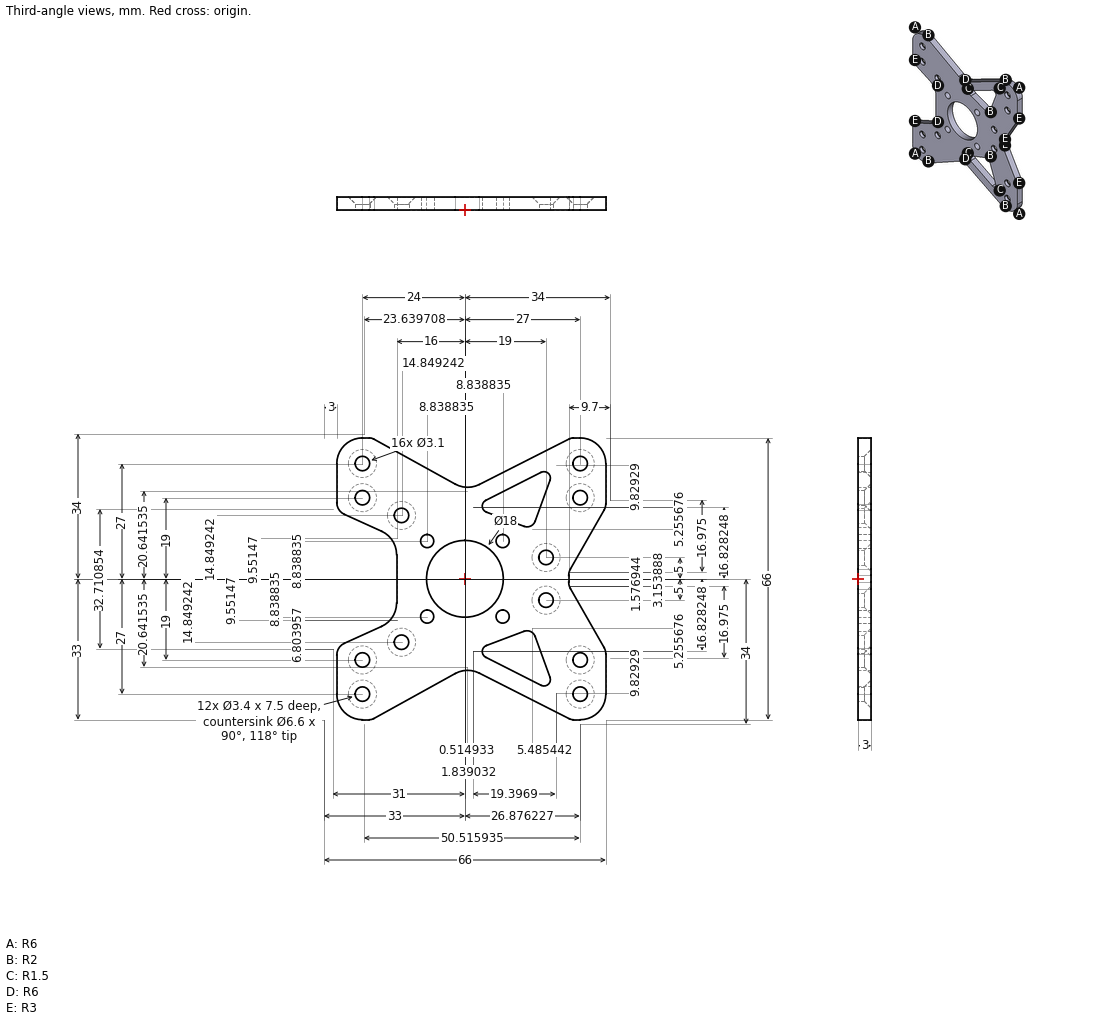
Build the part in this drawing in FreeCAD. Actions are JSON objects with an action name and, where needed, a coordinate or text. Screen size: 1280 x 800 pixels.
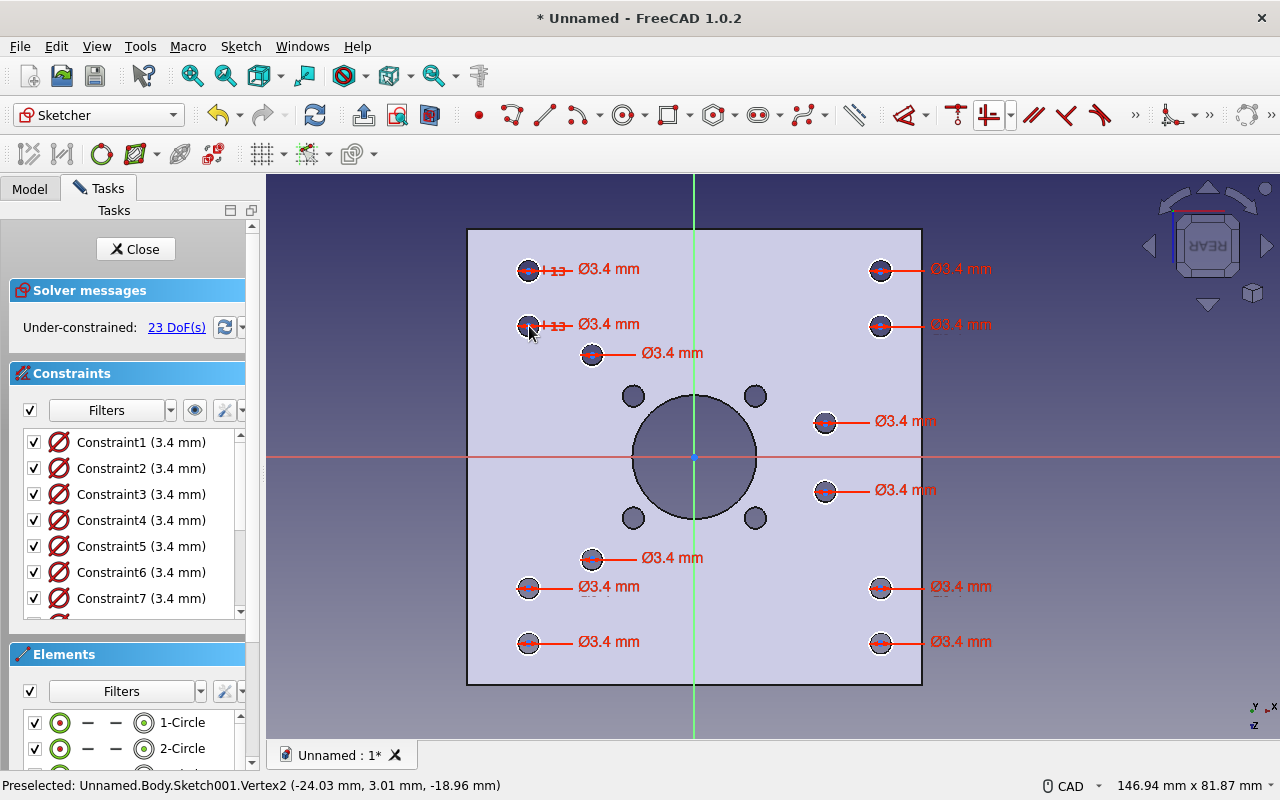
{"action": "left_click", "coordinate": [529, 326]}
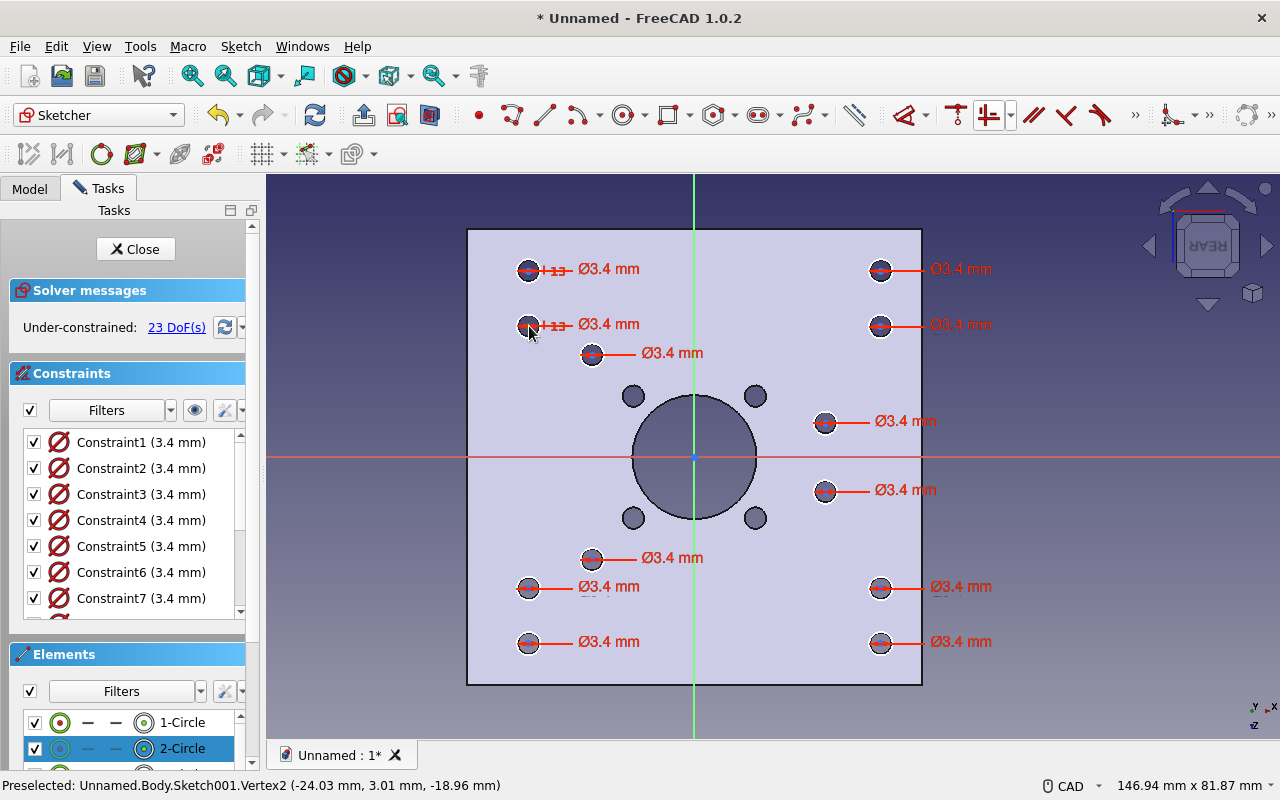
{"action": "left_click", "coordinate": [529, 589]}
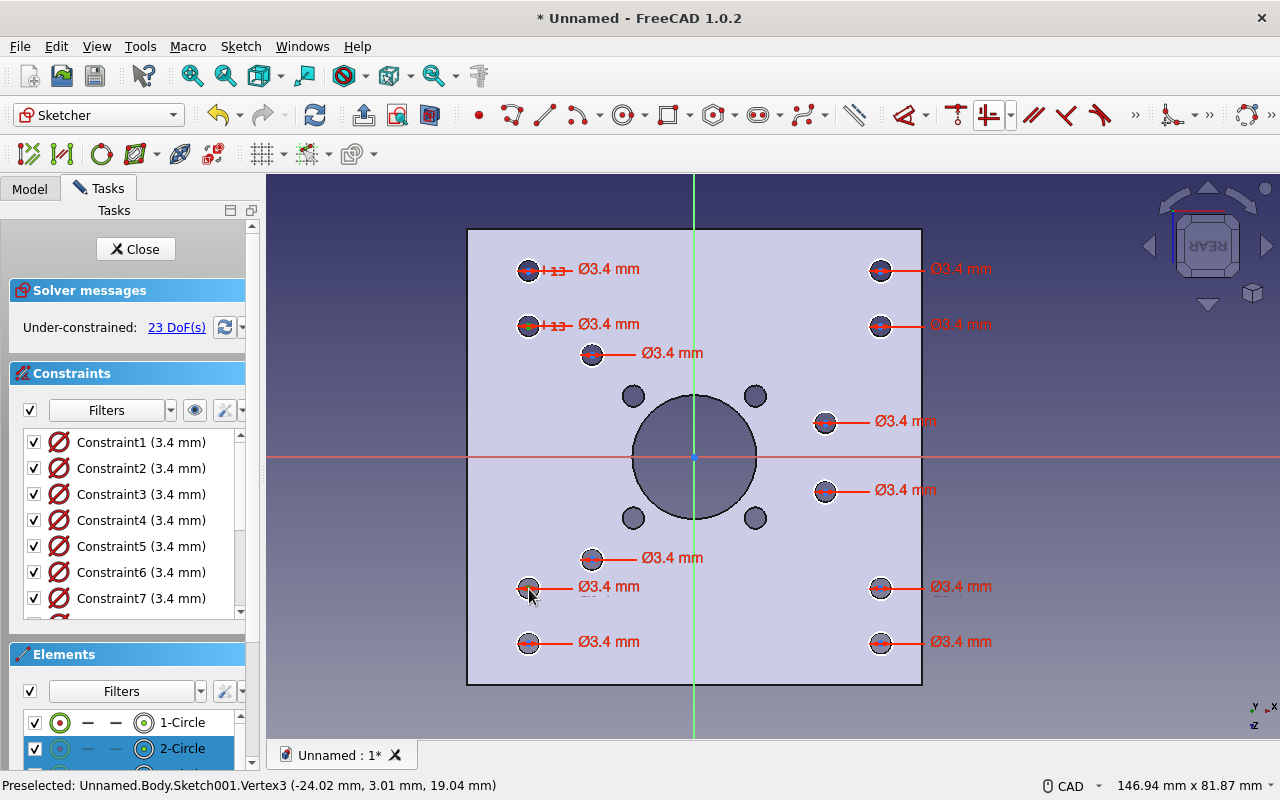
{"action": "left_click", "coordinate": [1010, 116]}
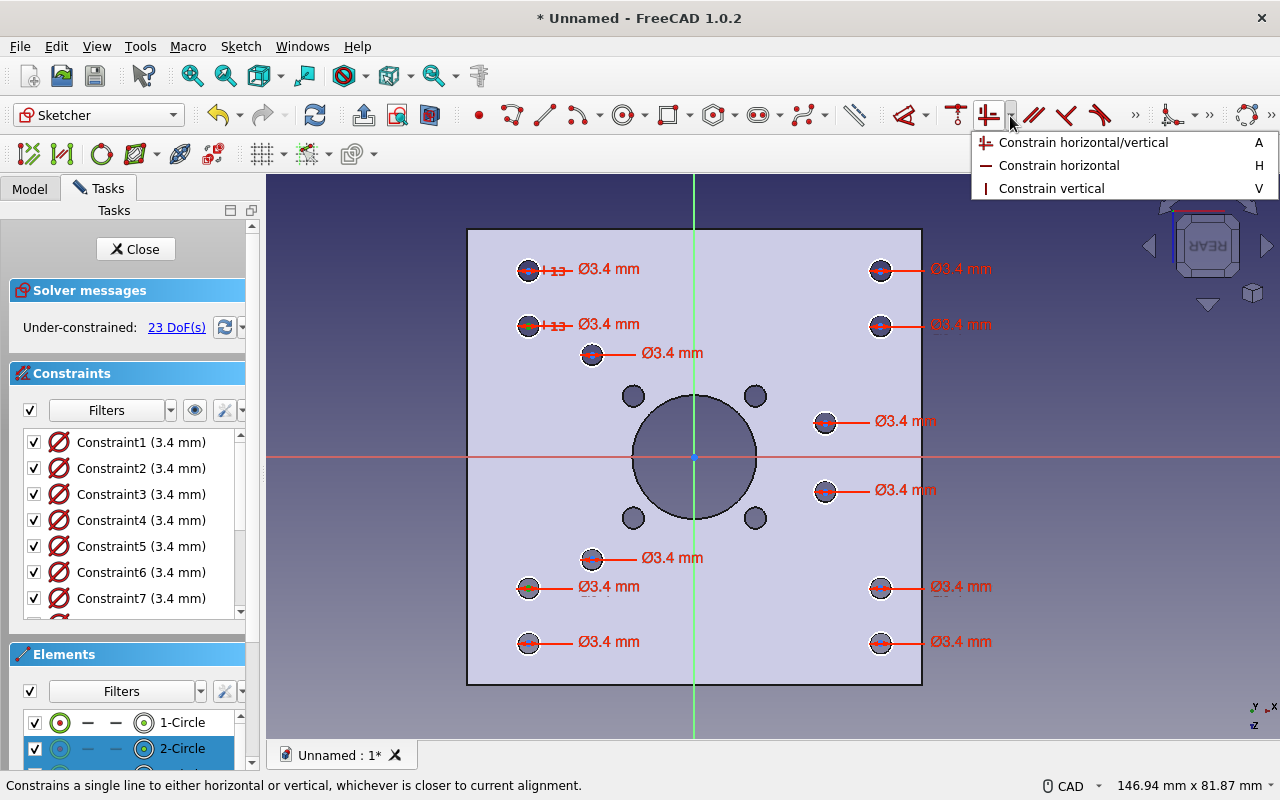
{"action": "left_click", "coordinate": [1125, 188]}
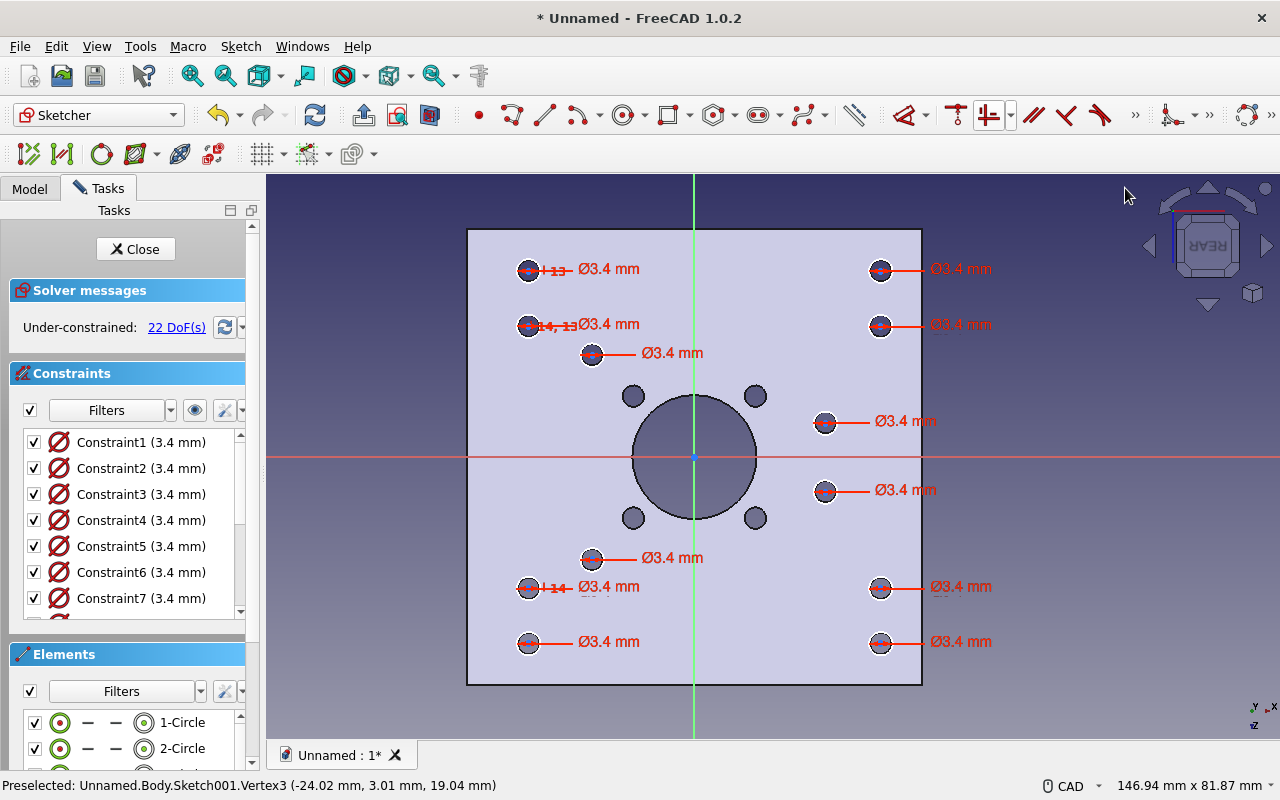
{"action": "left_click", "coordinate": [529, 589]}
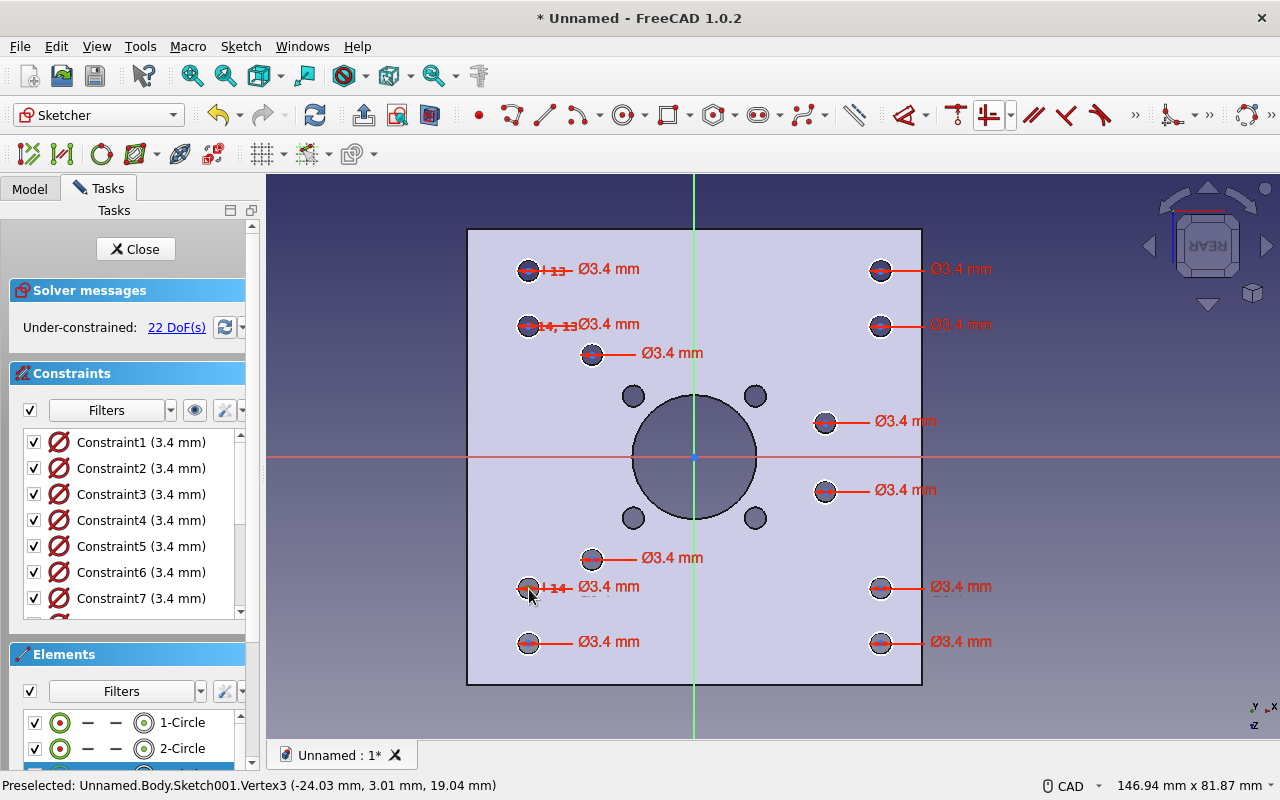
{"action": "left_click", "coordinate": [529, 644]}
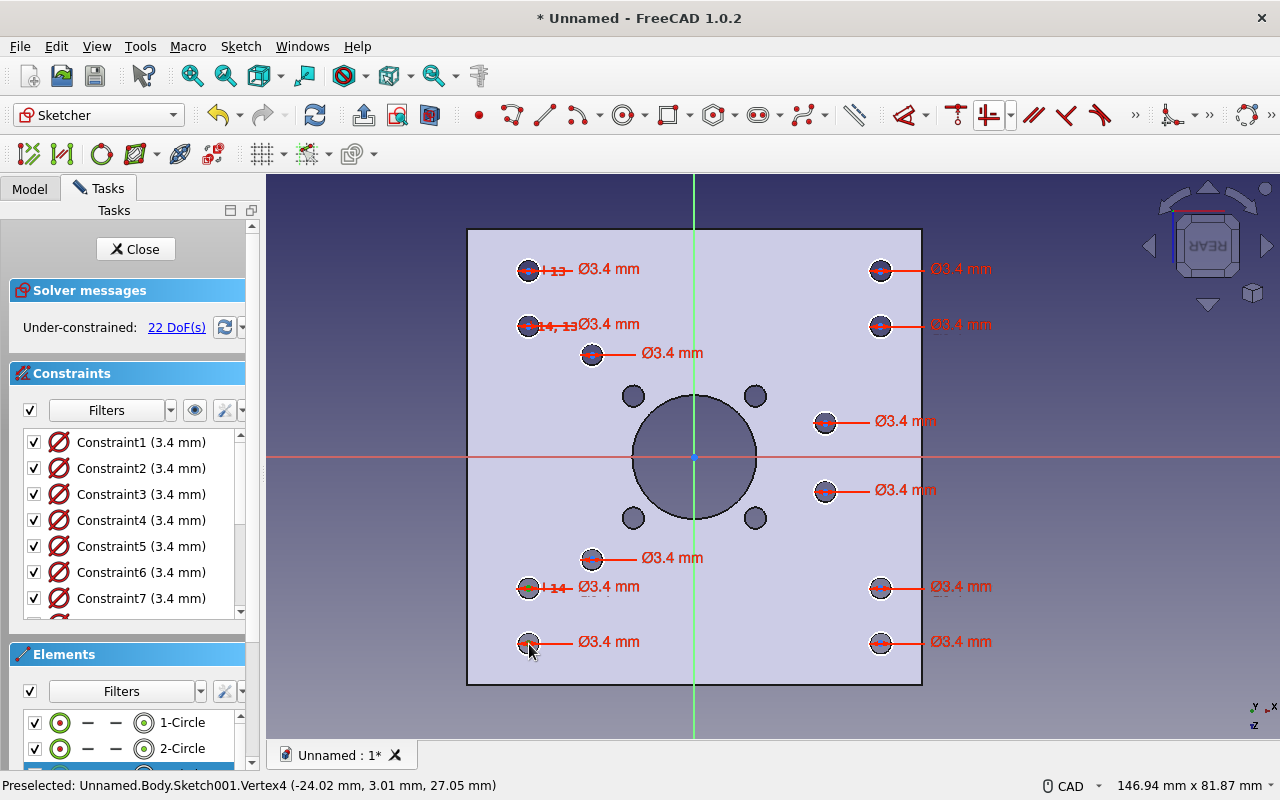
{"action": "left_click", "coordinate": [1010, 116]}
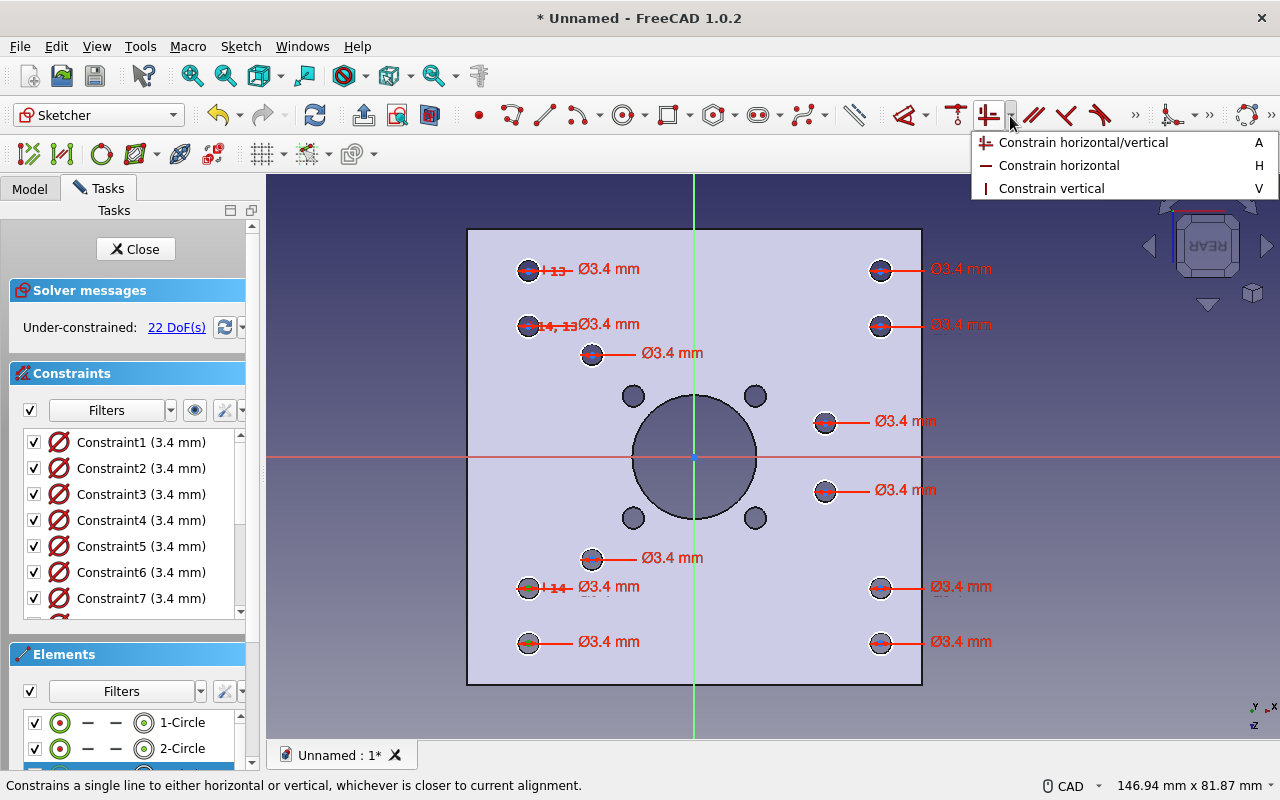
{"action": "left_click", "coordinate": [1125, 188]}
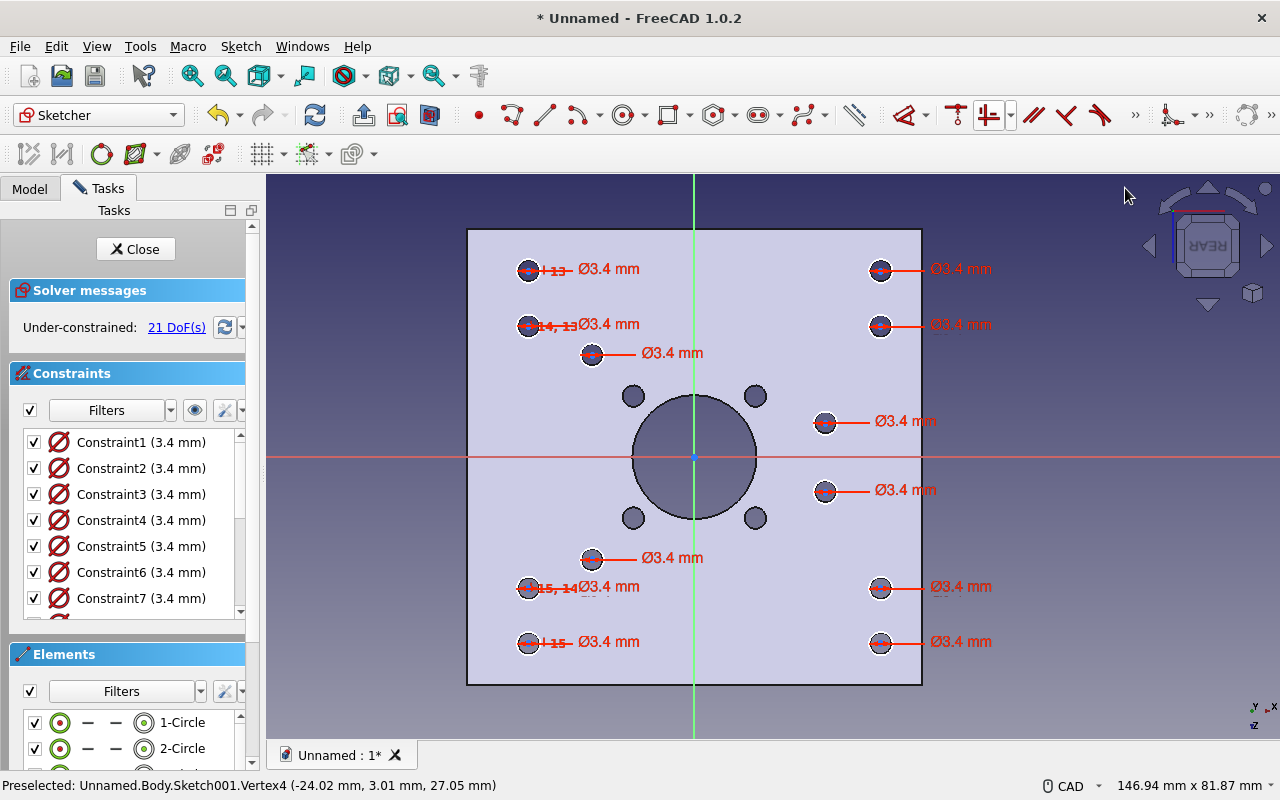
{"action": "left_click", "coordinate": [592, 355]}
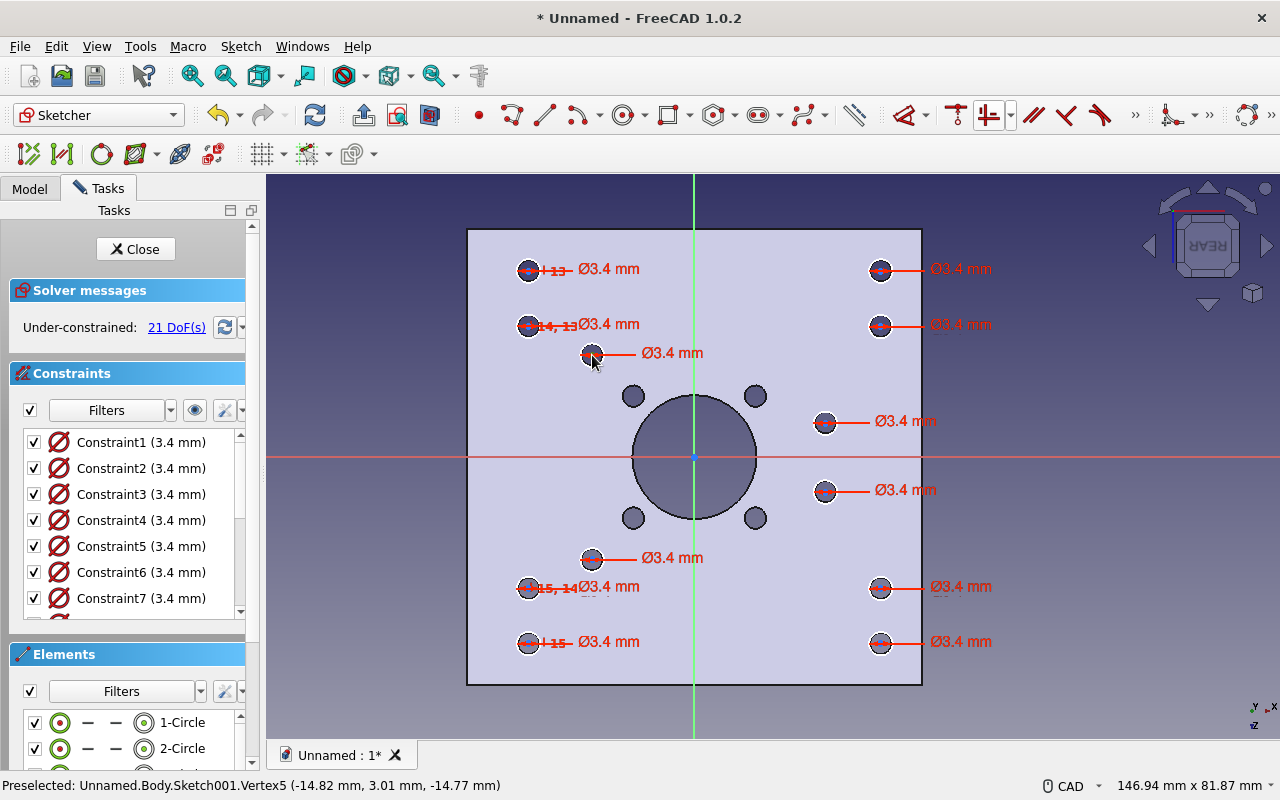
{"action": "left_click", "coordinate": [592, 560]}